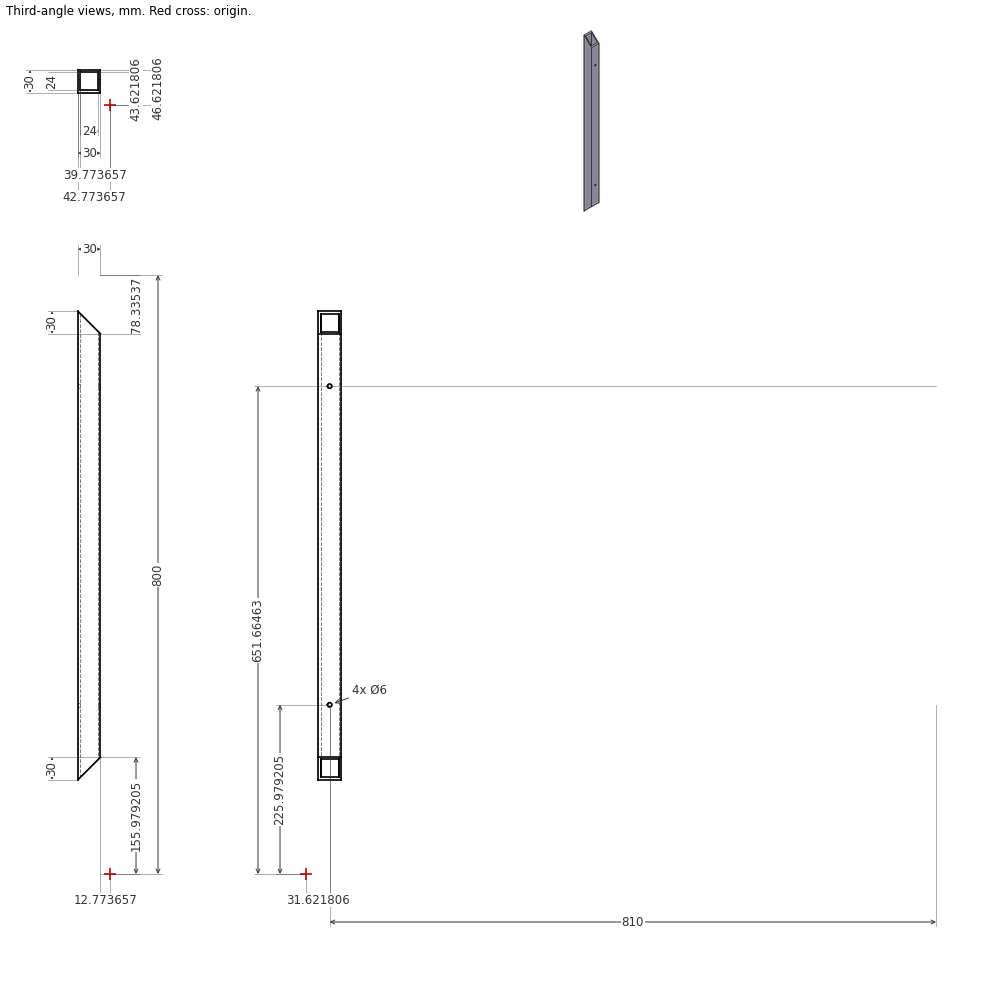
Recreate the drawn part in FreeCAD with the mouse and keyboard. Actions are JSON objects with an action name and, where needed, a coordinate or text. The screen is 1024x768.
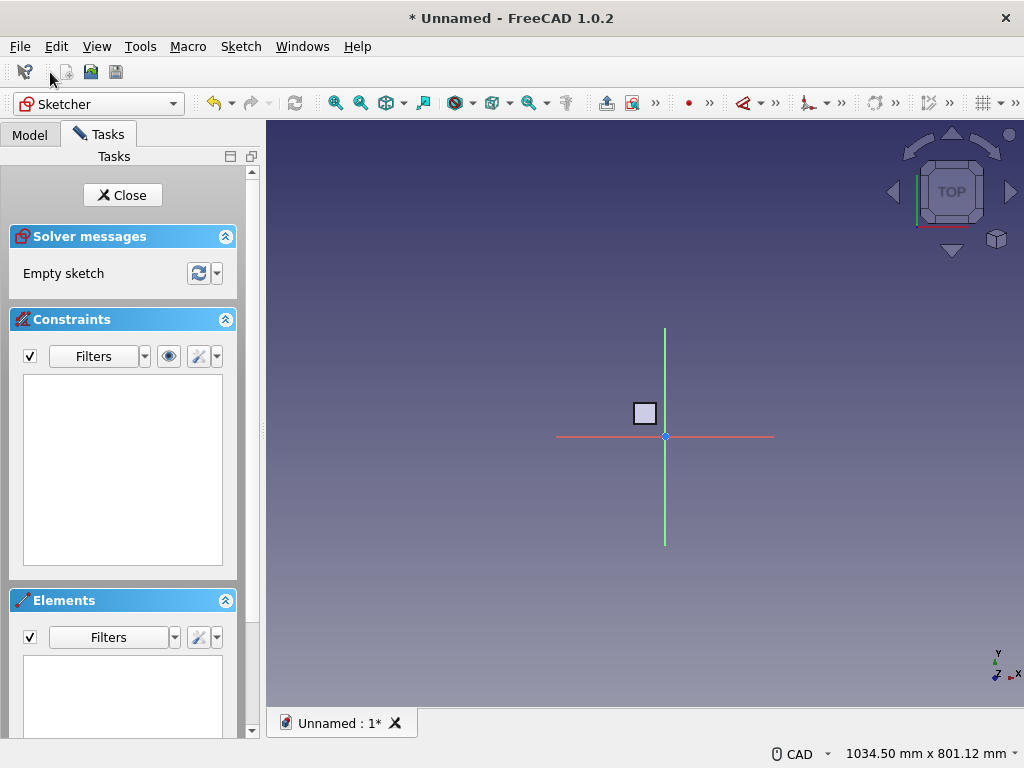
{"action": "scroll", "coordinate": [658, 421], "scroll_direction": "up", "scroll_amount": 12}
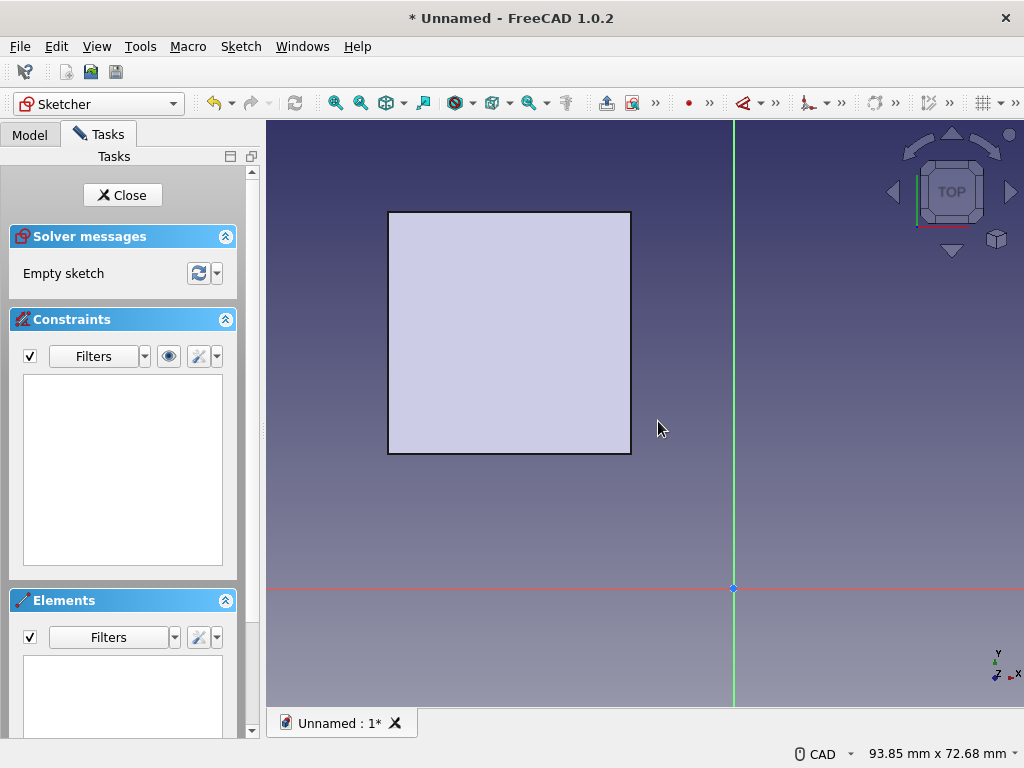
{"action": "key", "text": "g r"}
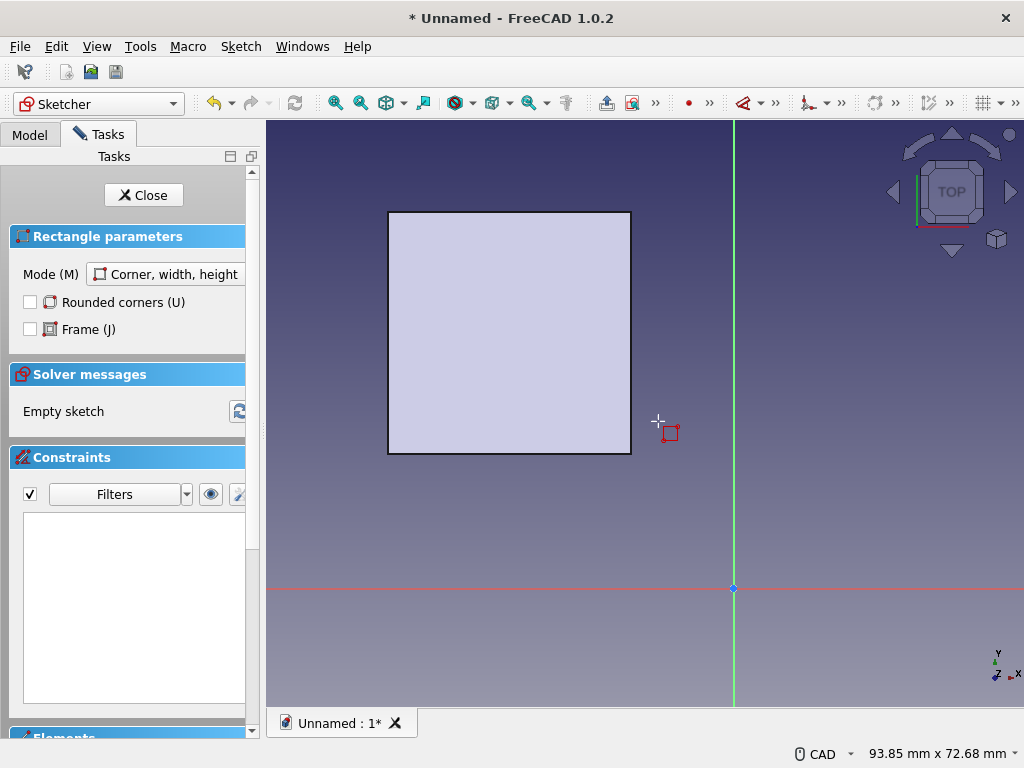
{"action": "left_click", "coordinate": [413, 236]}
{"action": "left_click", "coordinate": [606, 430]}
{"action": "key", "text": "Escape"}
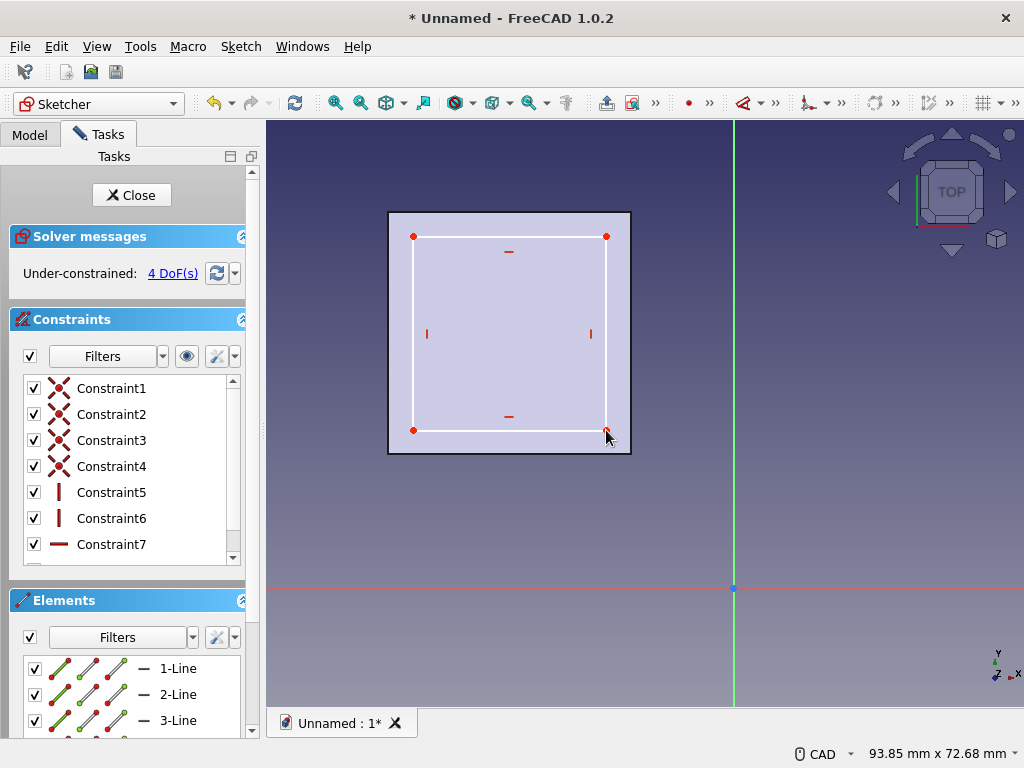
{"action": "left_click", "coordinate": [742, 104]}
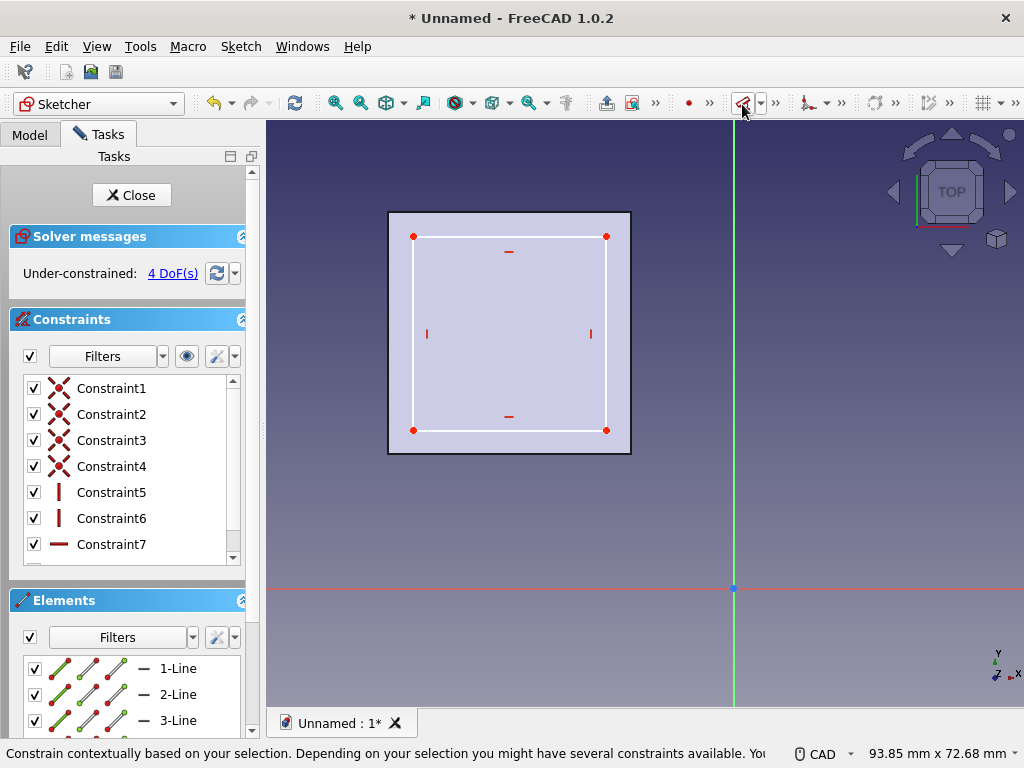
{"action": "left_click", "coordinate": [413, 295]}
{"action": "left_click", "coordinate": [379, 334]}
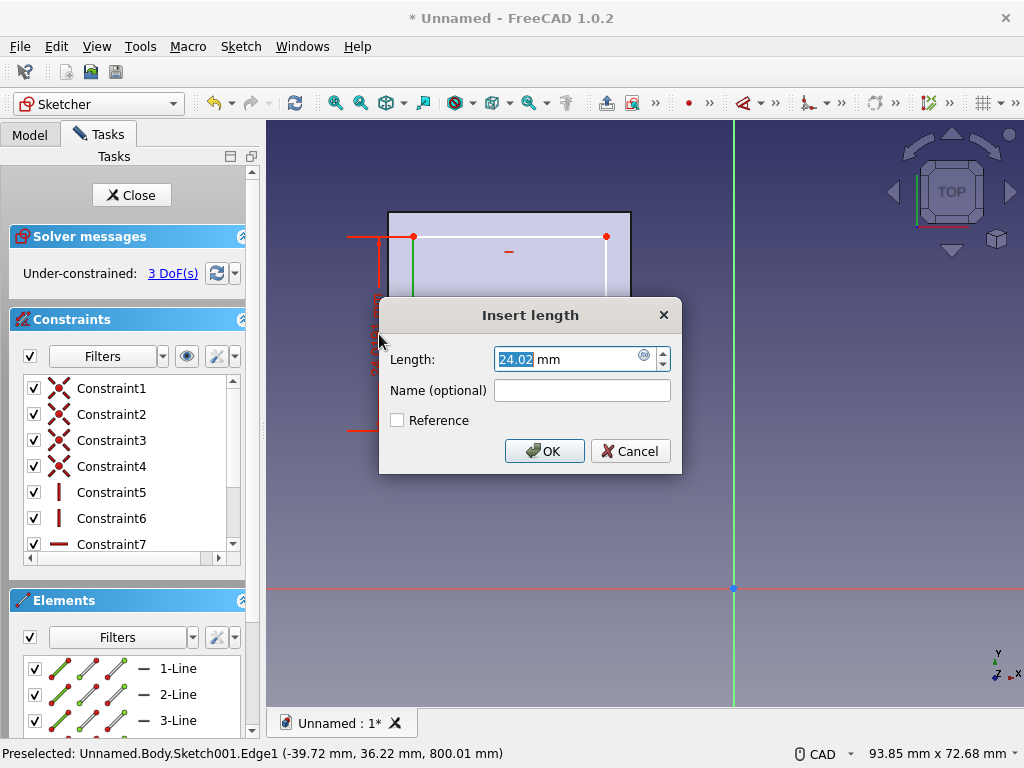
{"action": "type", "text": "24"}
{"action": "key", "text": "Return"}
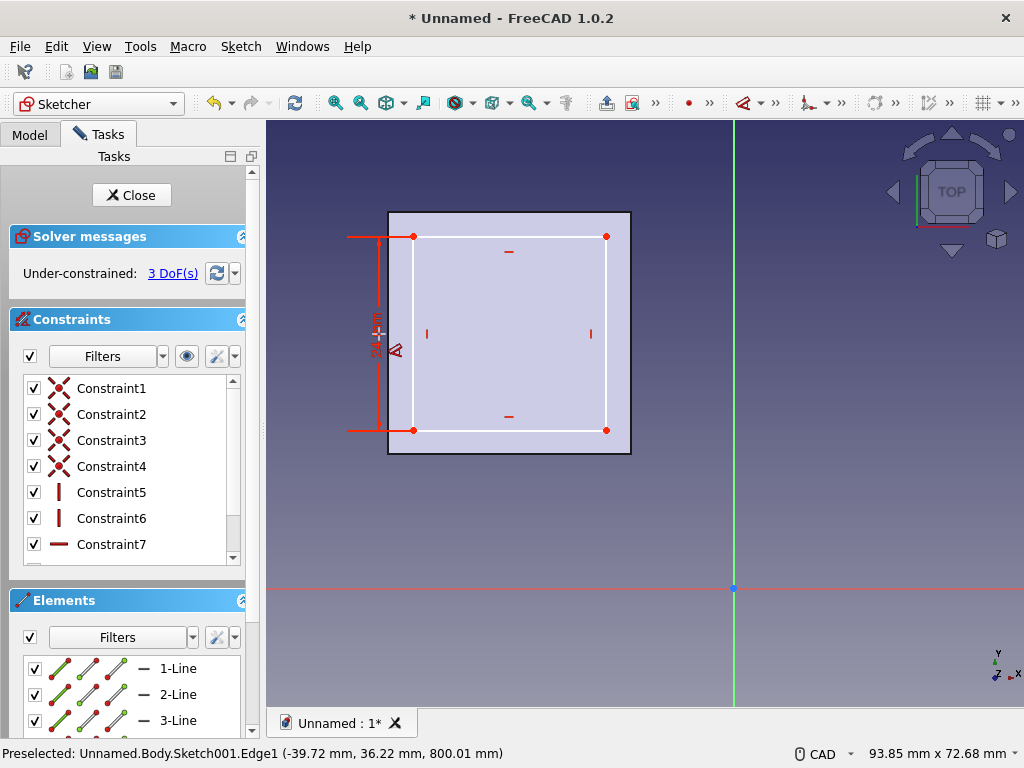
{"action": "left_click", "coordinate": [471, 431]}
{"action": "left_click", "coordinate": [510, 465]}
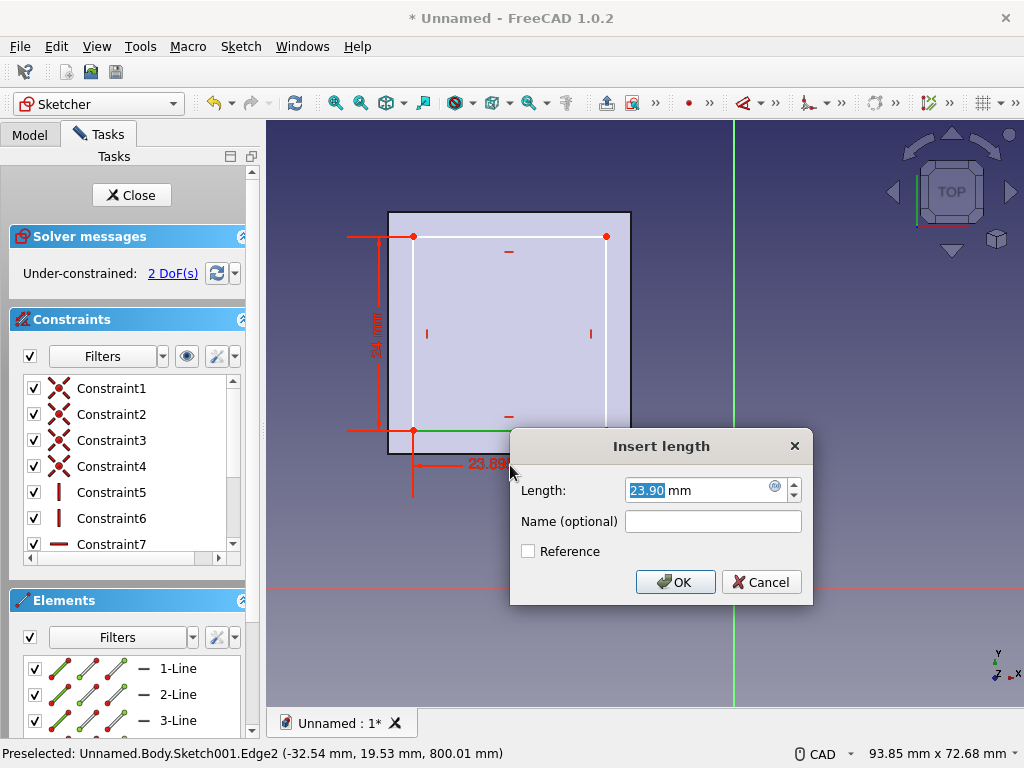
{"action": "type", "text": "24"}
{"action": "key", "text": "Return"}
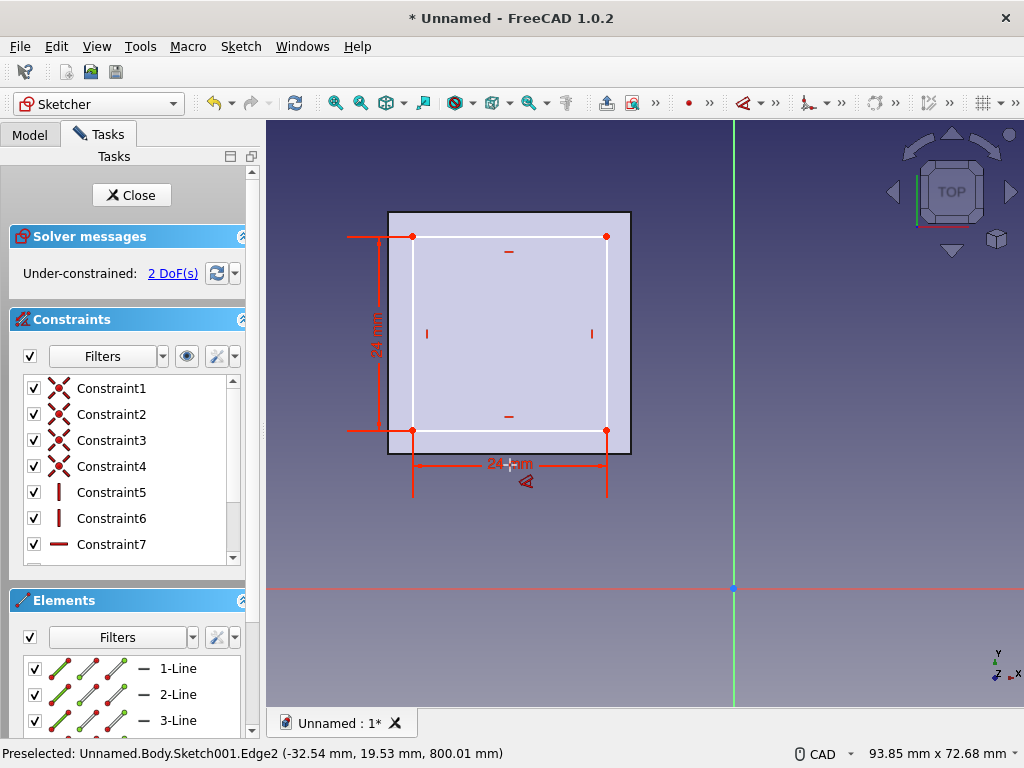
{"action": "left_click", "coordinate": [413, 237]}
{"action": "left_click", "coordinate": [573, 623]}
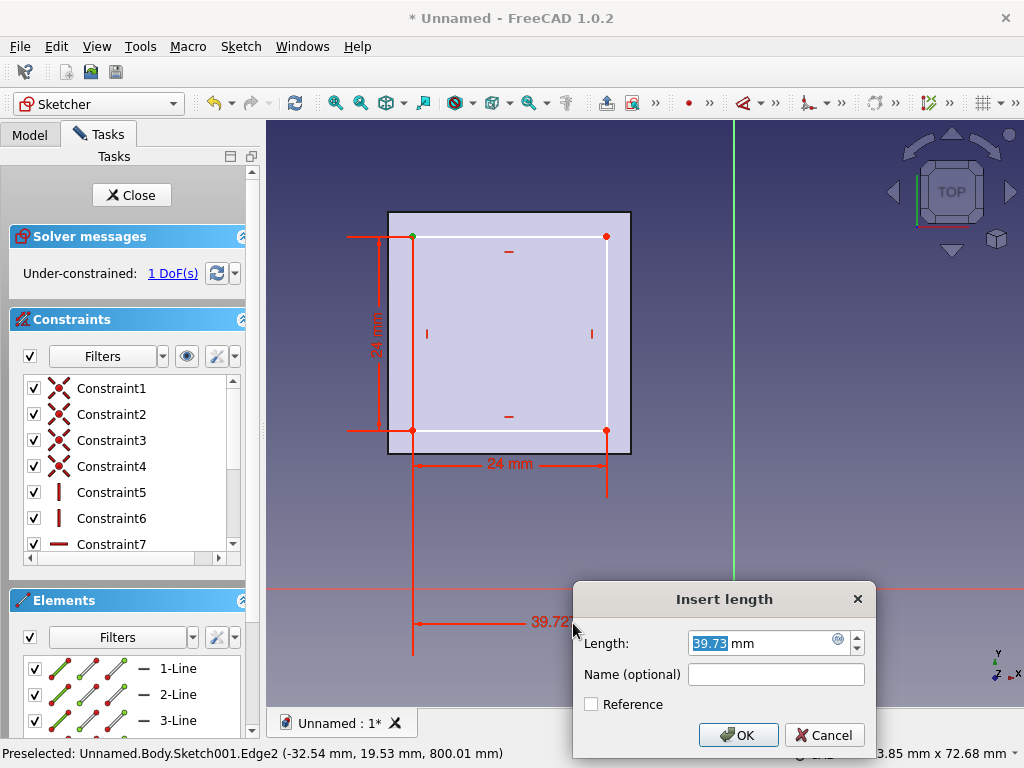
{"action": "type", "text": "39.773657"}
{"action": "key", "text": "Return"}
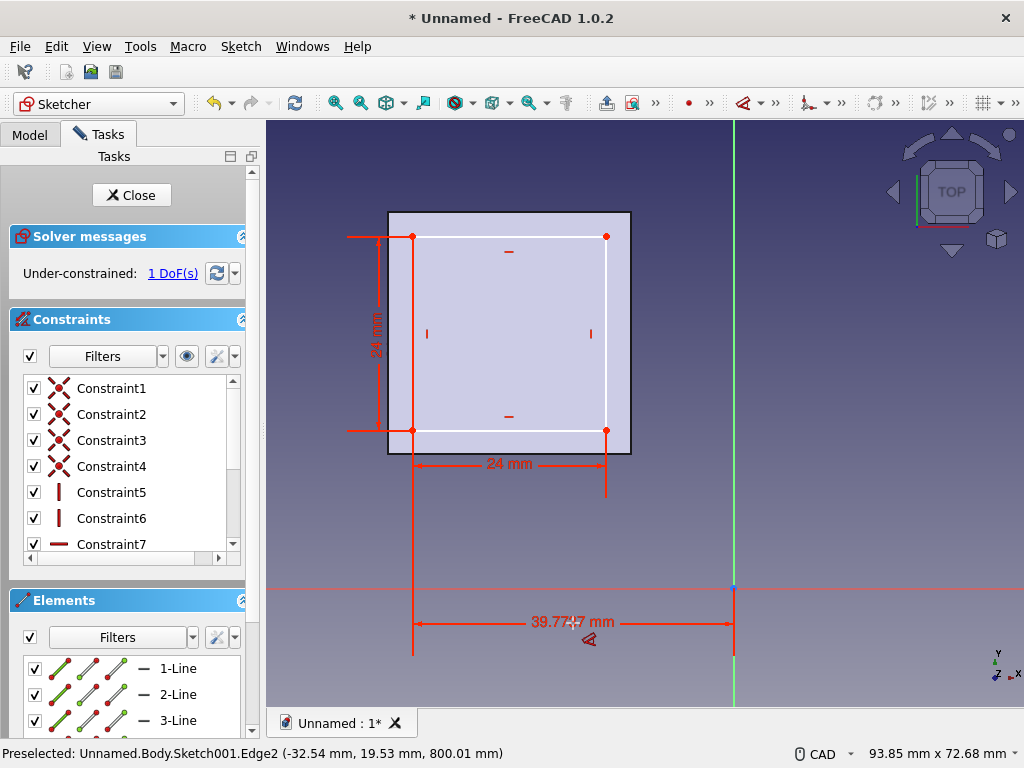
{"action": "left_click", "coordinate": [413, 237]}
{"action": "left_click", "coordinate": [379, 413]}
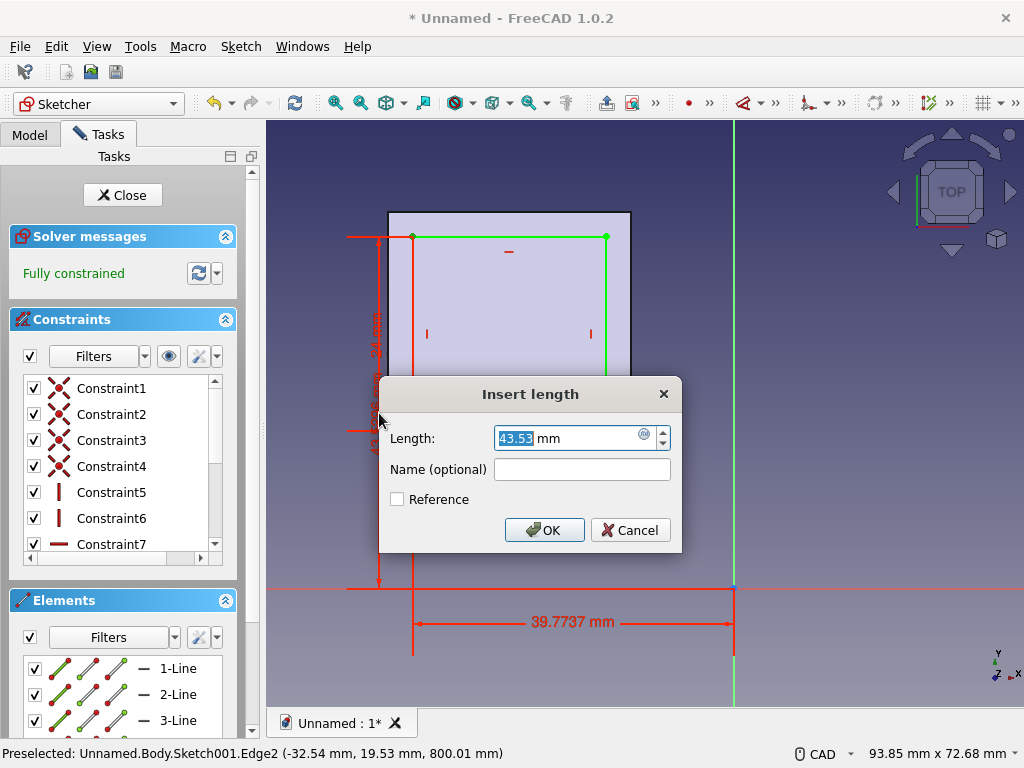
{"action": "type", "text": "43.621806"}
{"action": "key", "text": "Return"}
{"action": "key", "text": "Escape"}